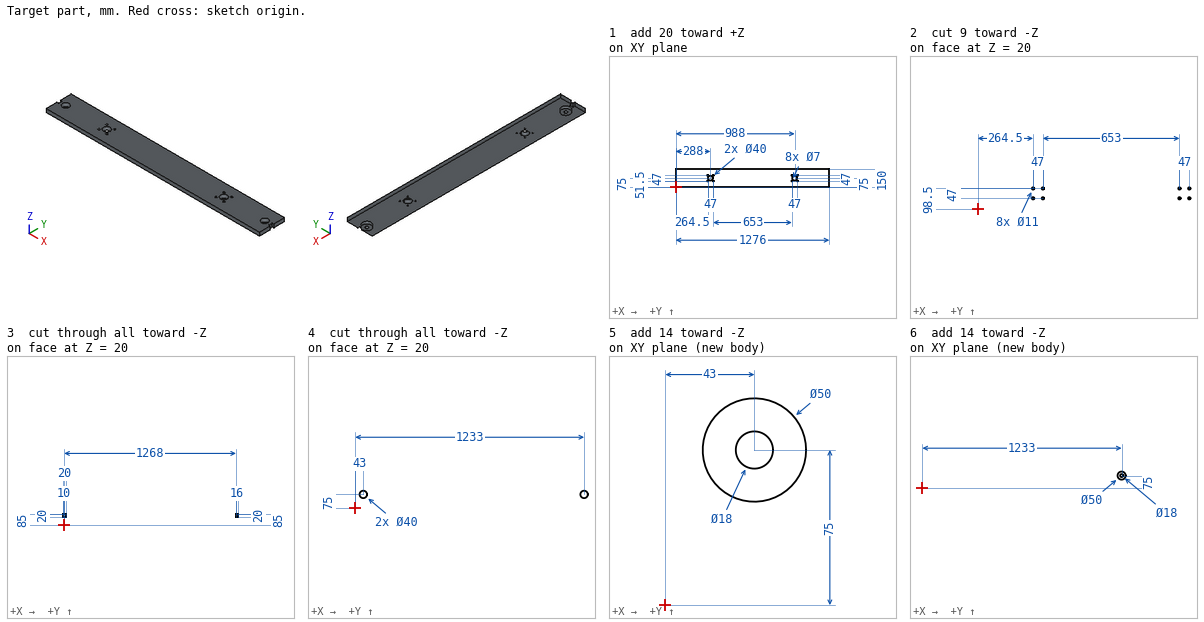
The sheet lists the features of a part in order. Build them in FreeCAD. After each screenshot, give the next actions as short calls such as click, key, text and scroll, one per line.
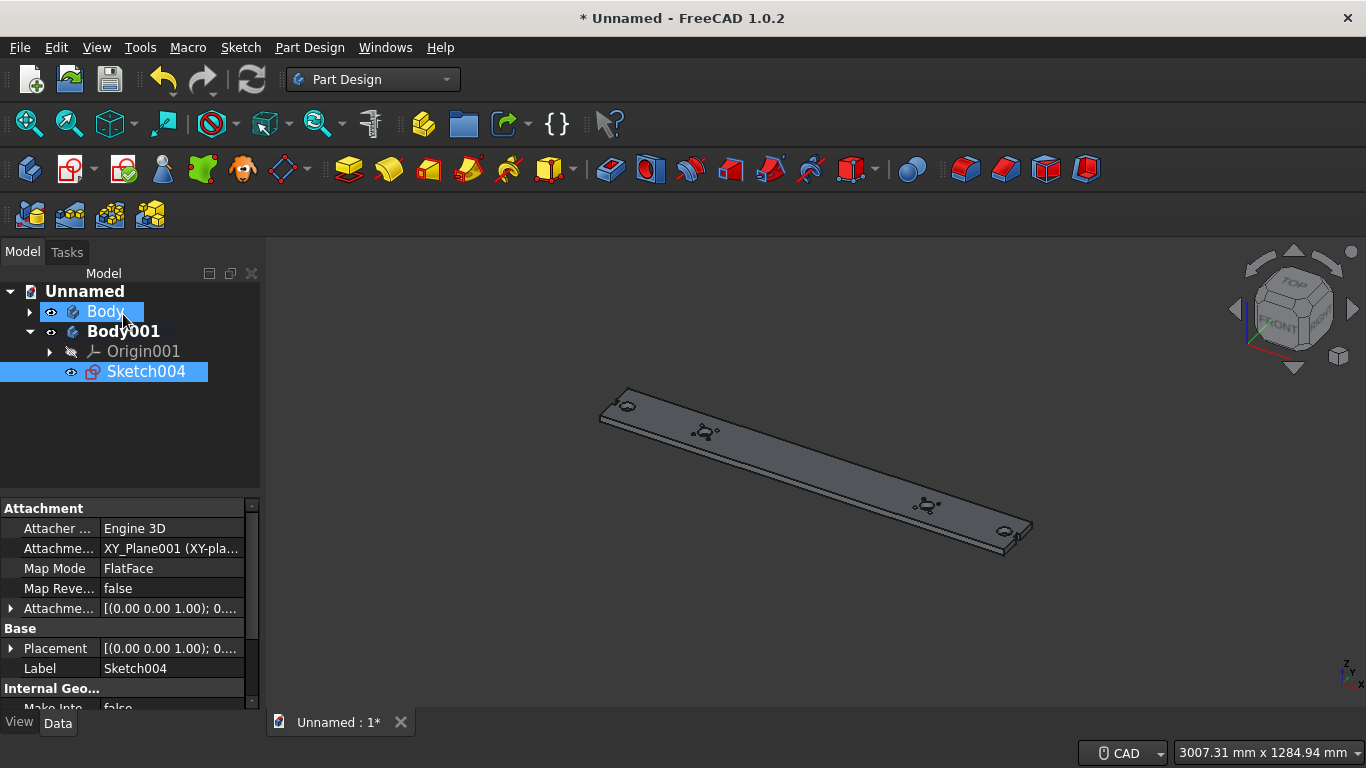
click(350, 170)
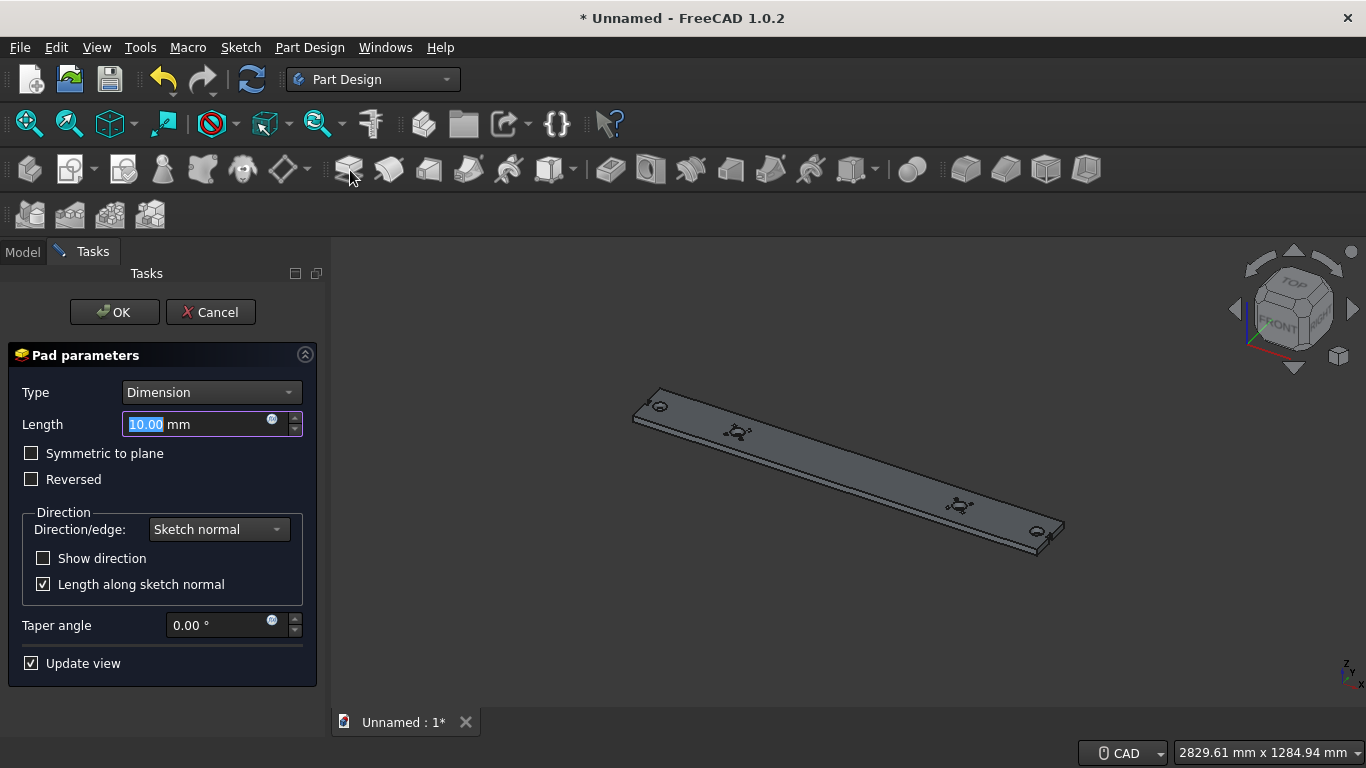
text(14)
key(Tab)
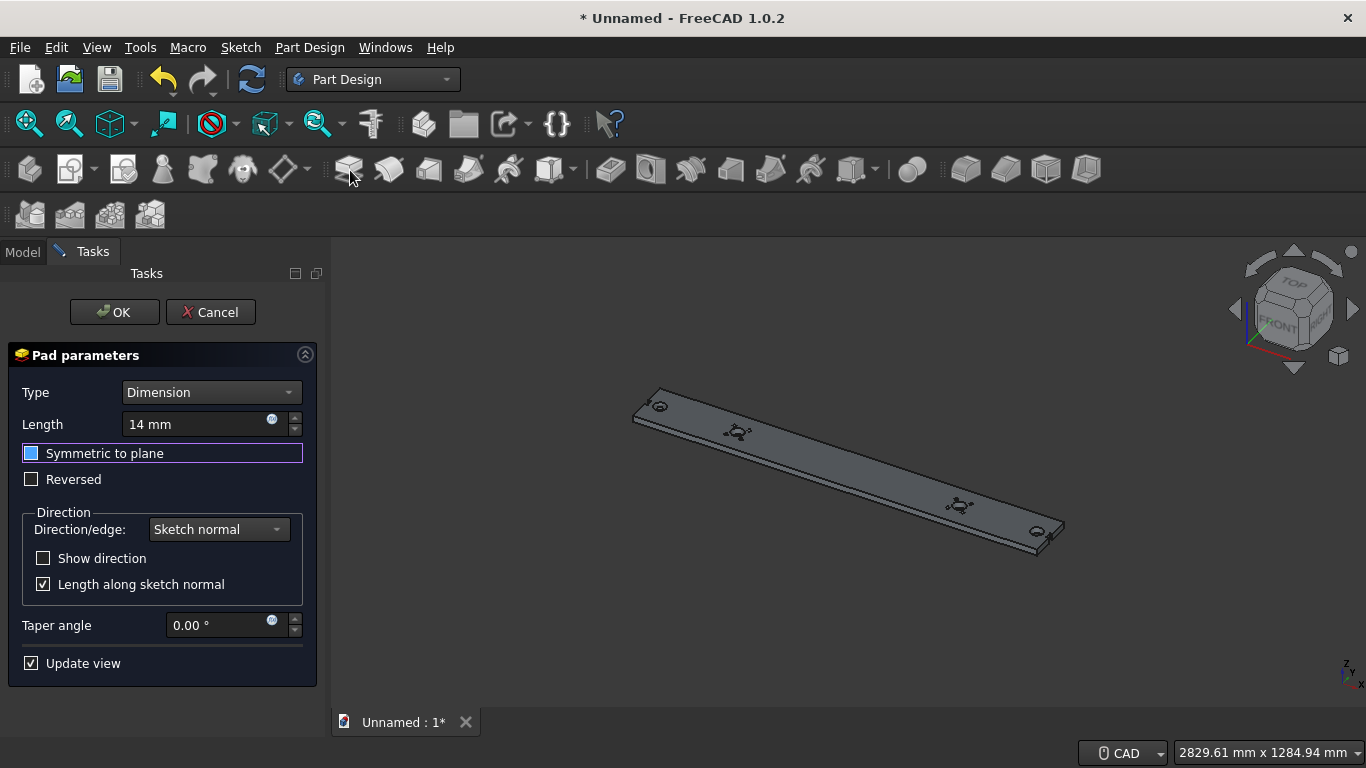
click(30, 479)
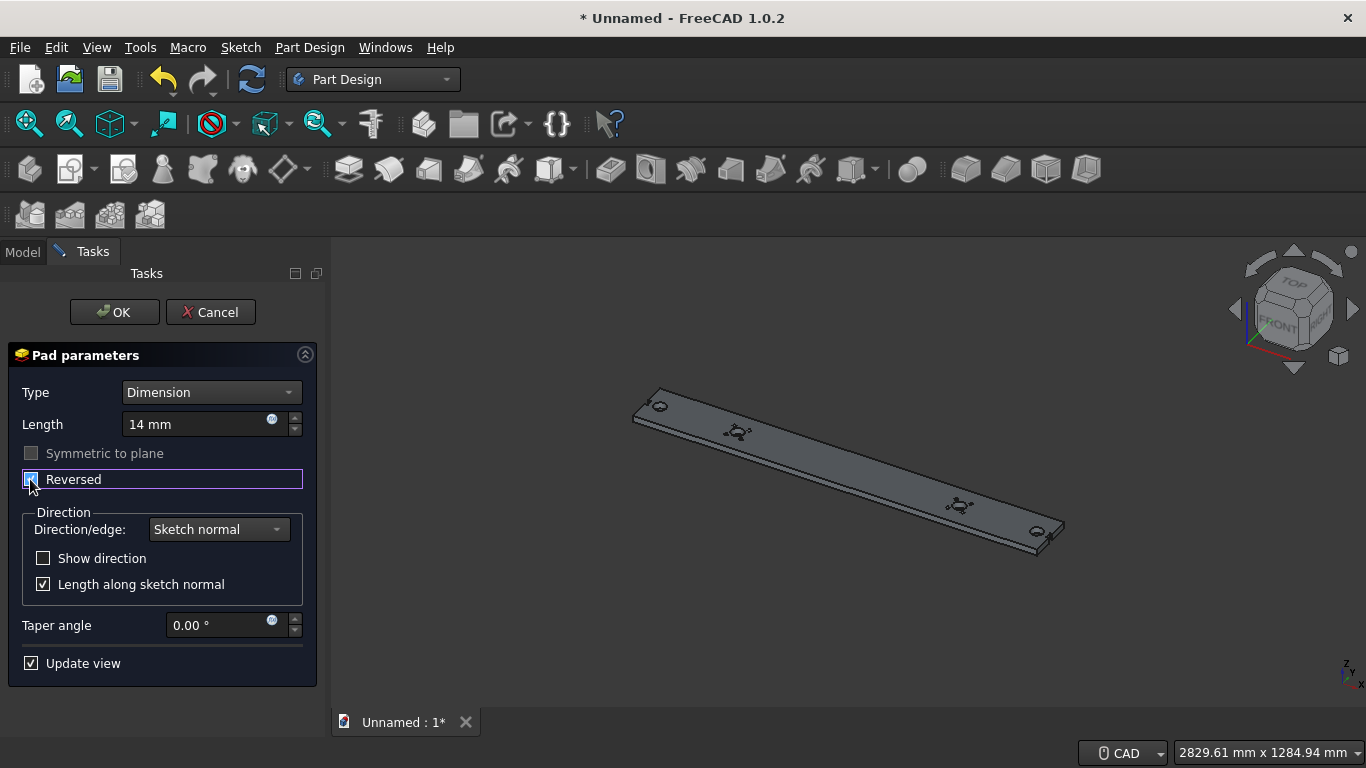
click(115, 312)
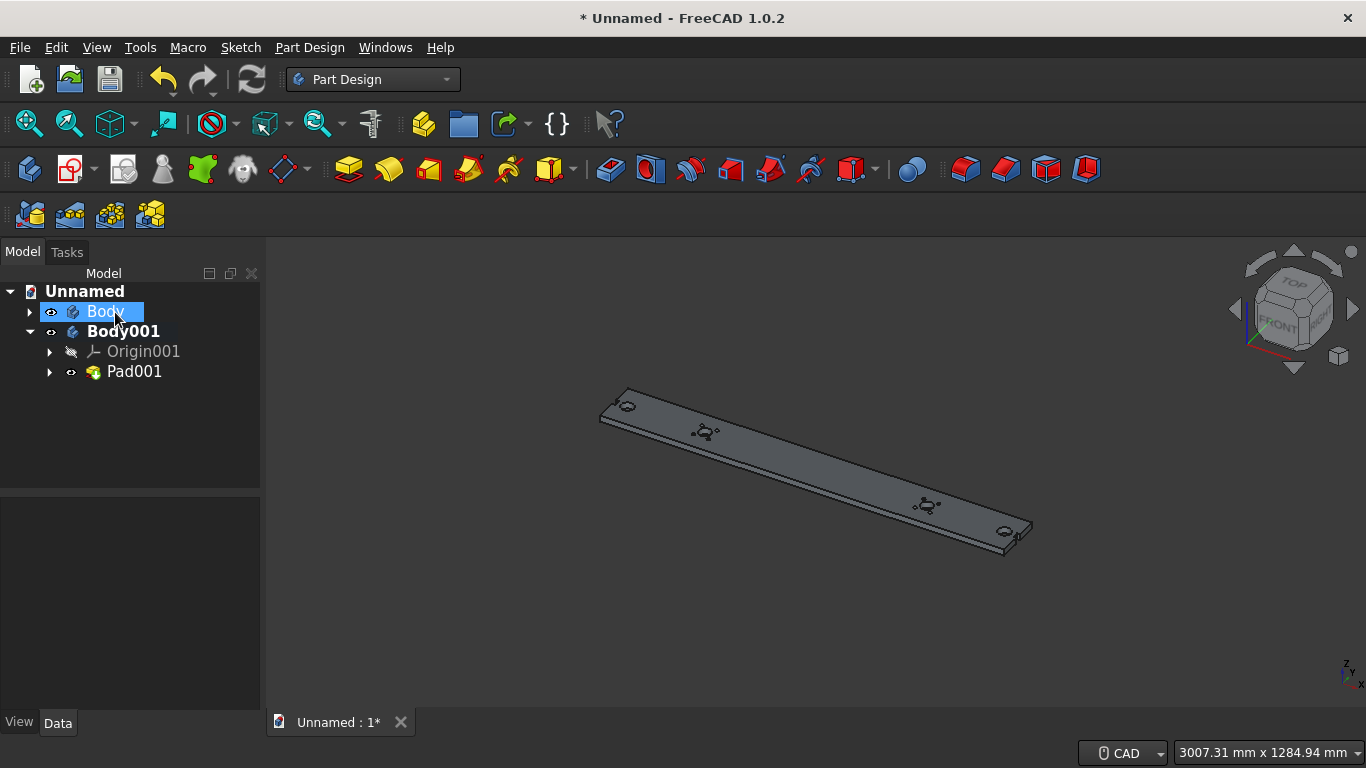
click(30, 124)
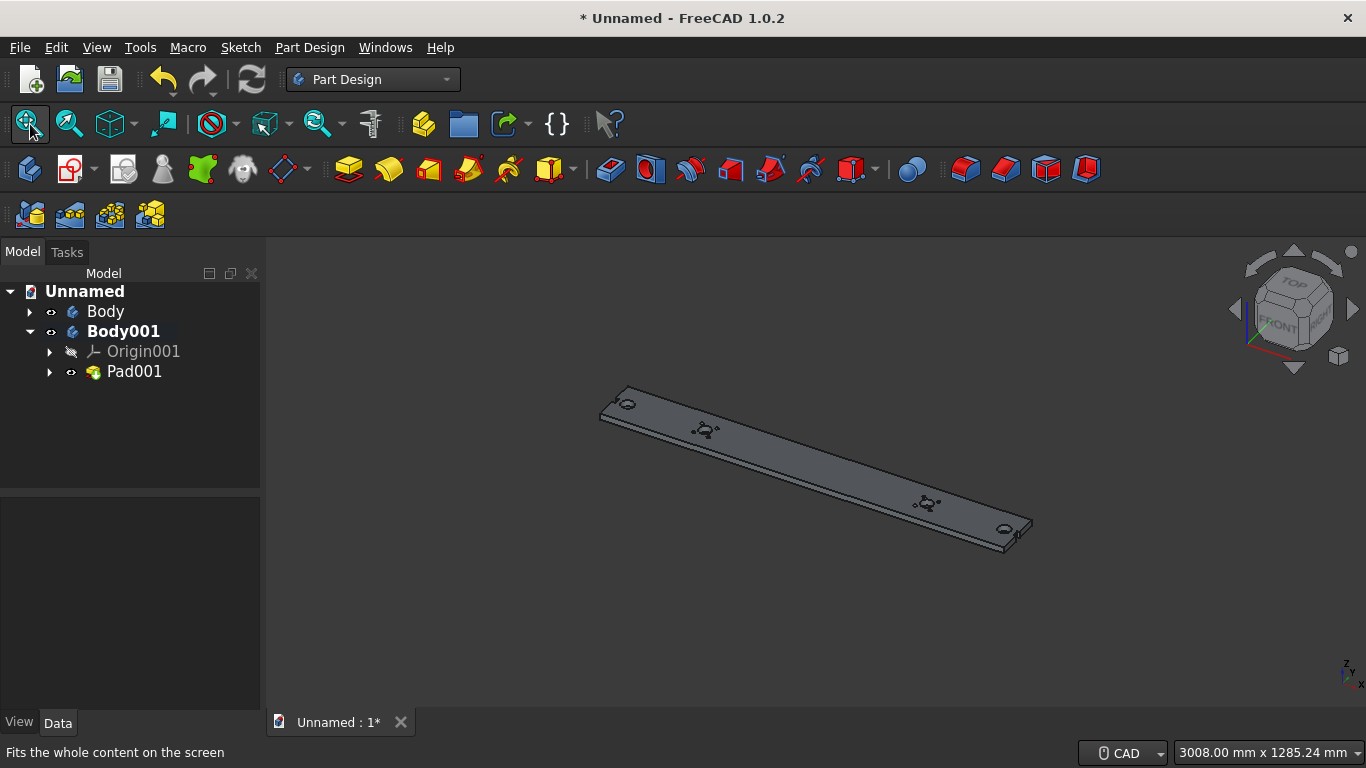
click(30, 170)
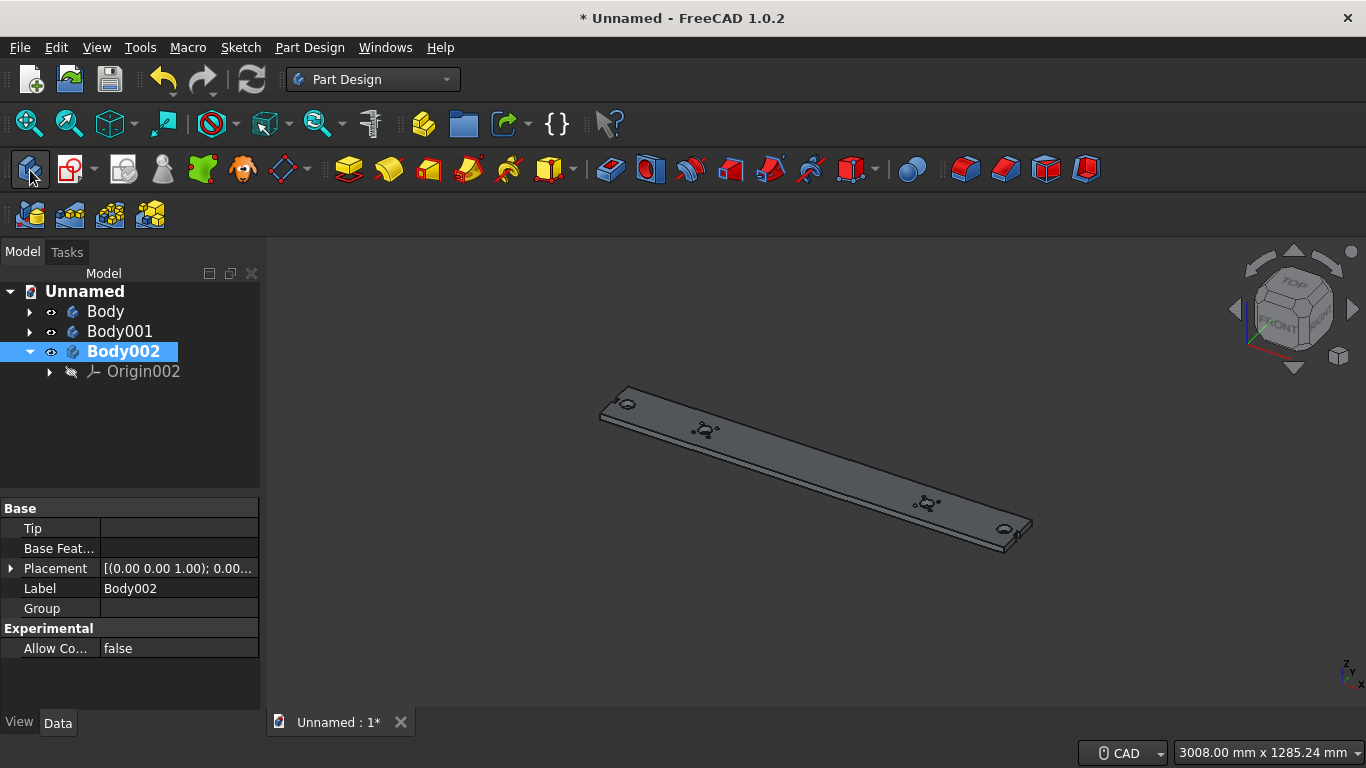
click(306, 667)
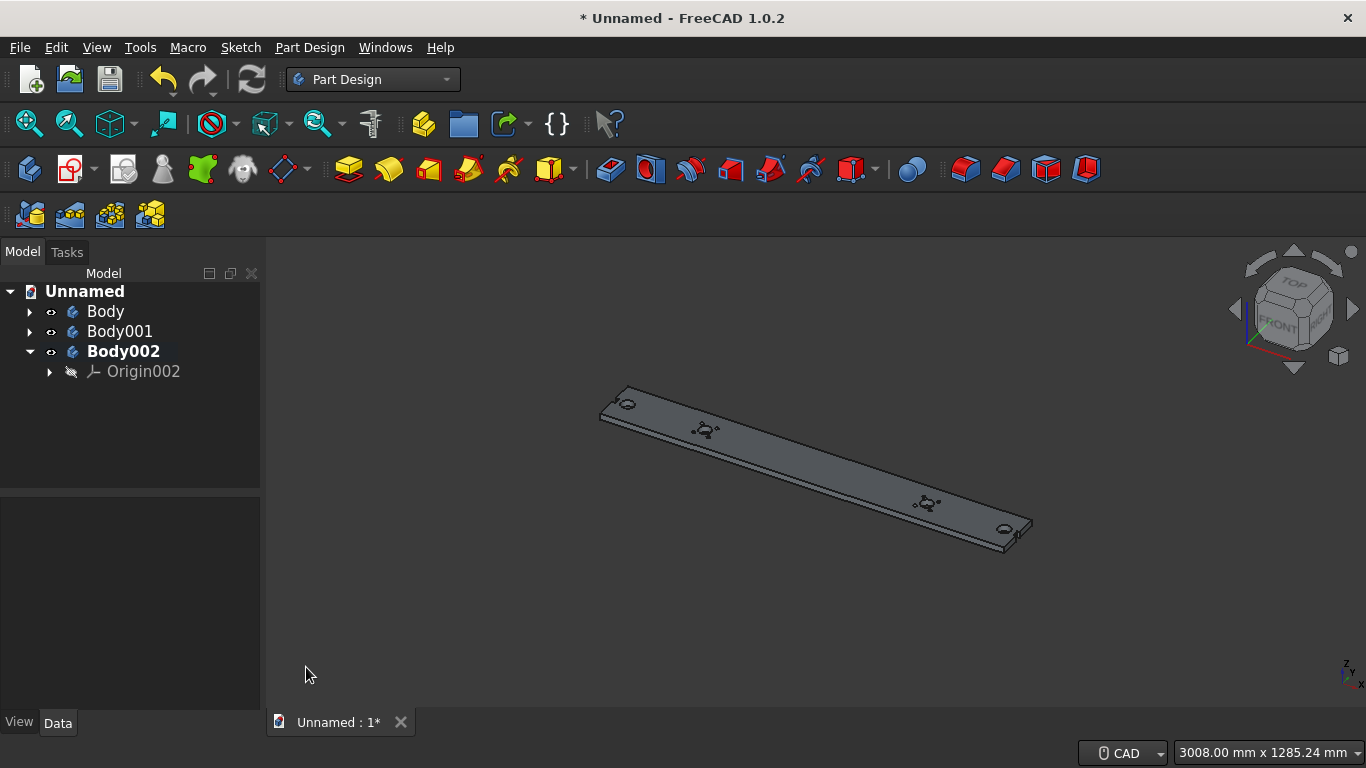
click(70, 170)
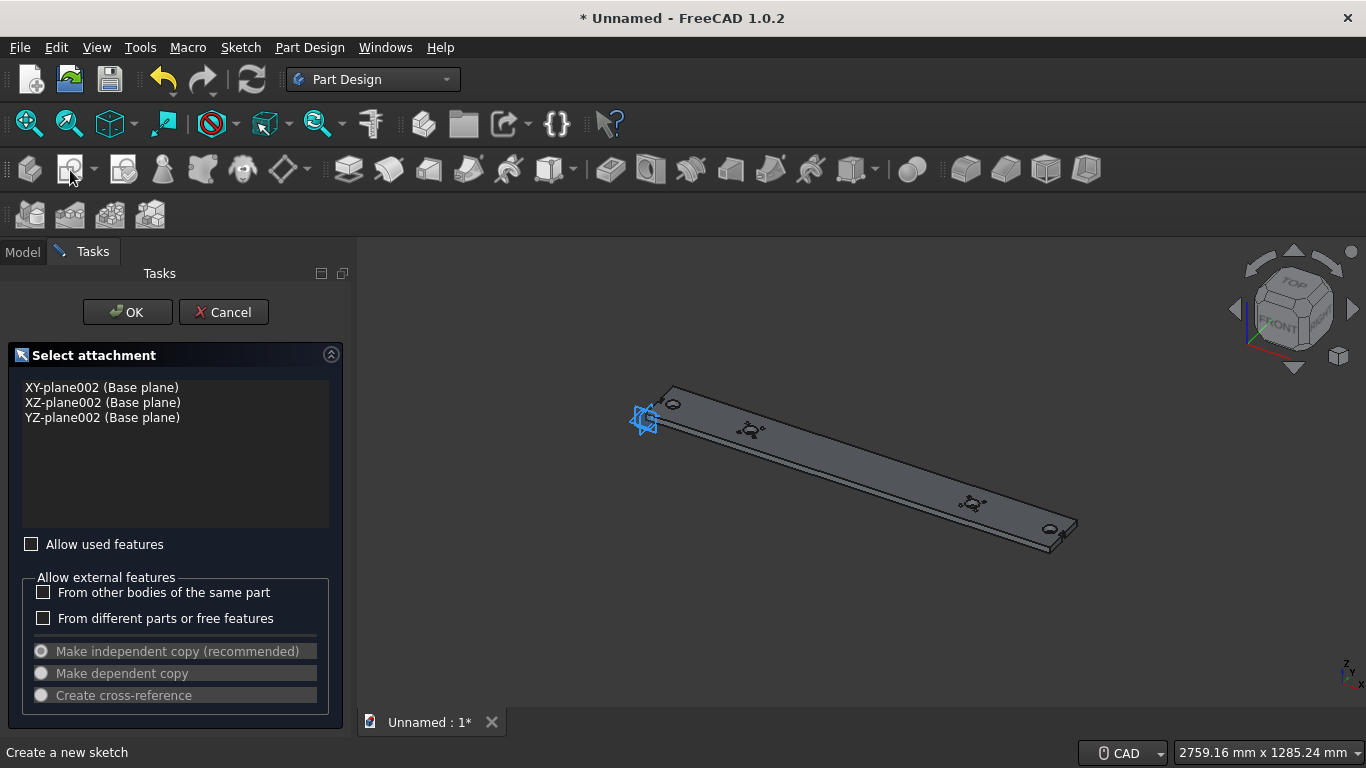
click(82, 388)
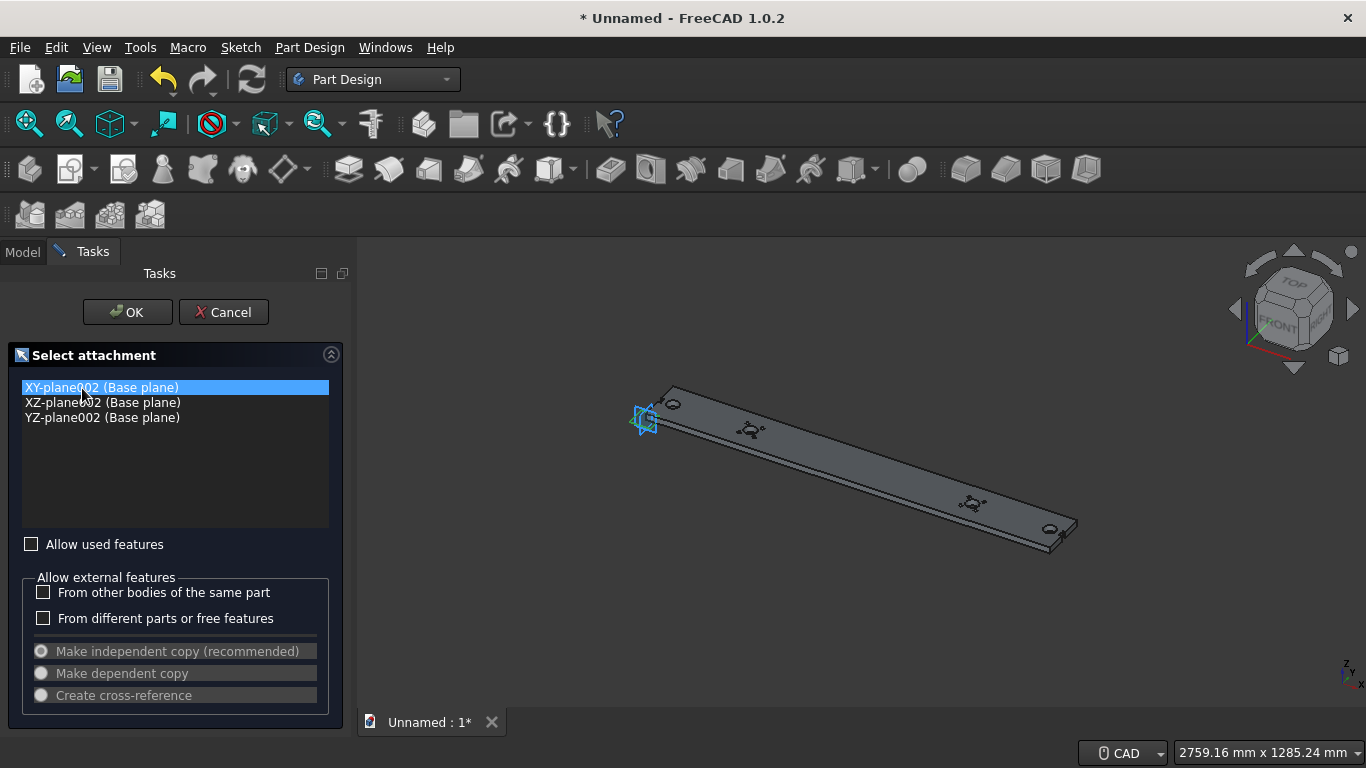
click(128, 312)